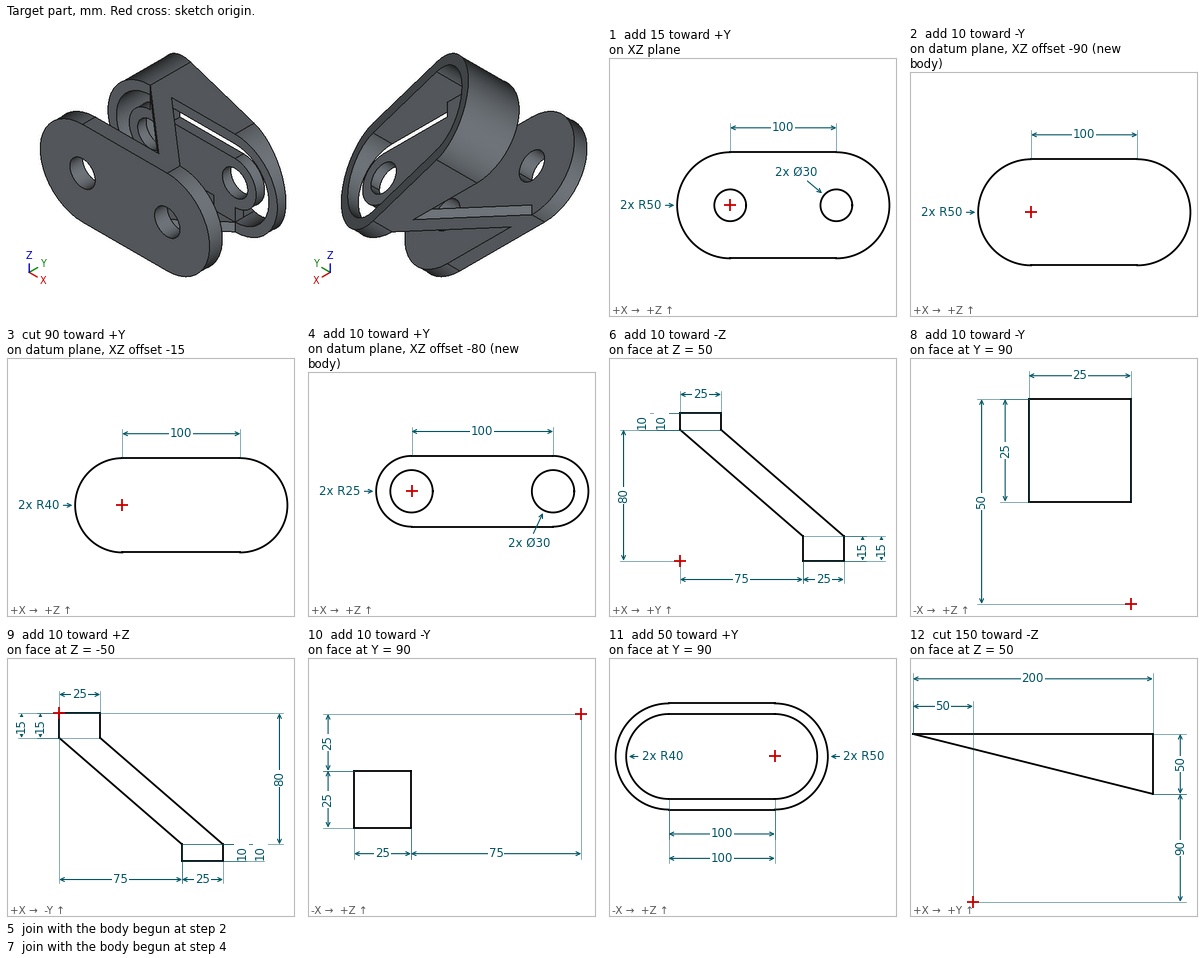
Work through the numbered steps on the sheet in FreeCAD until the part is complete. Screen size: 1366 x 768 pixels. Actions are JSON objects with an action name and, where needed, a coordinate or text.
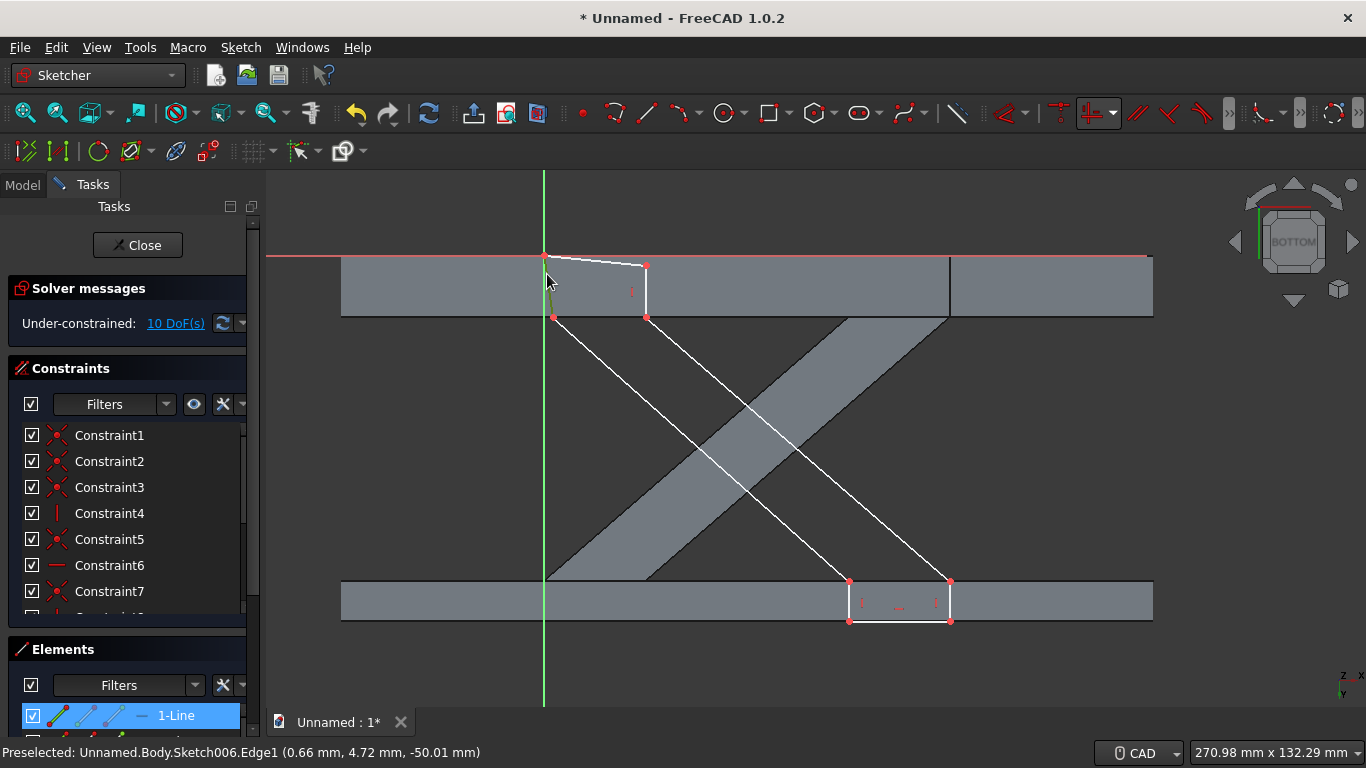
{"action": "left_click", "coordinate": [1116, 114]}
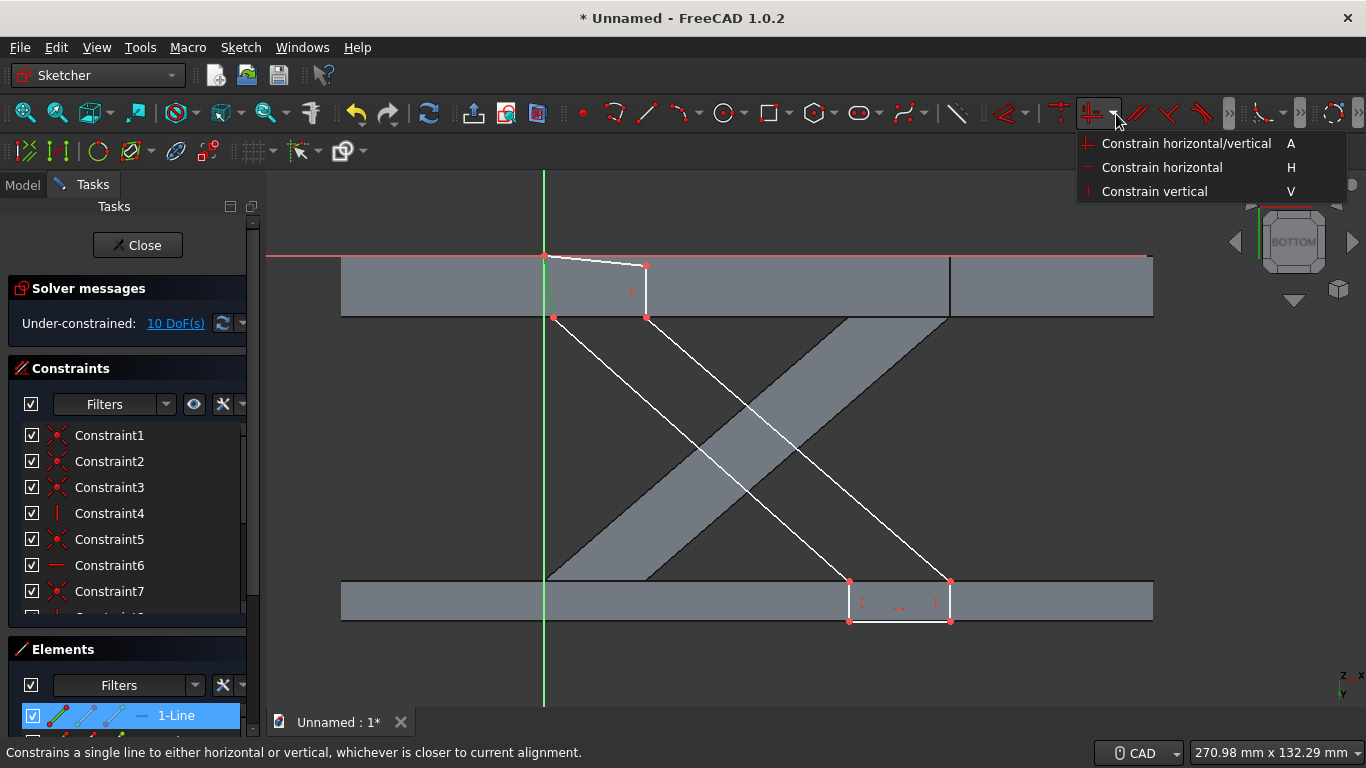
{"action": "left_click", "coordinate": [1212, 191]}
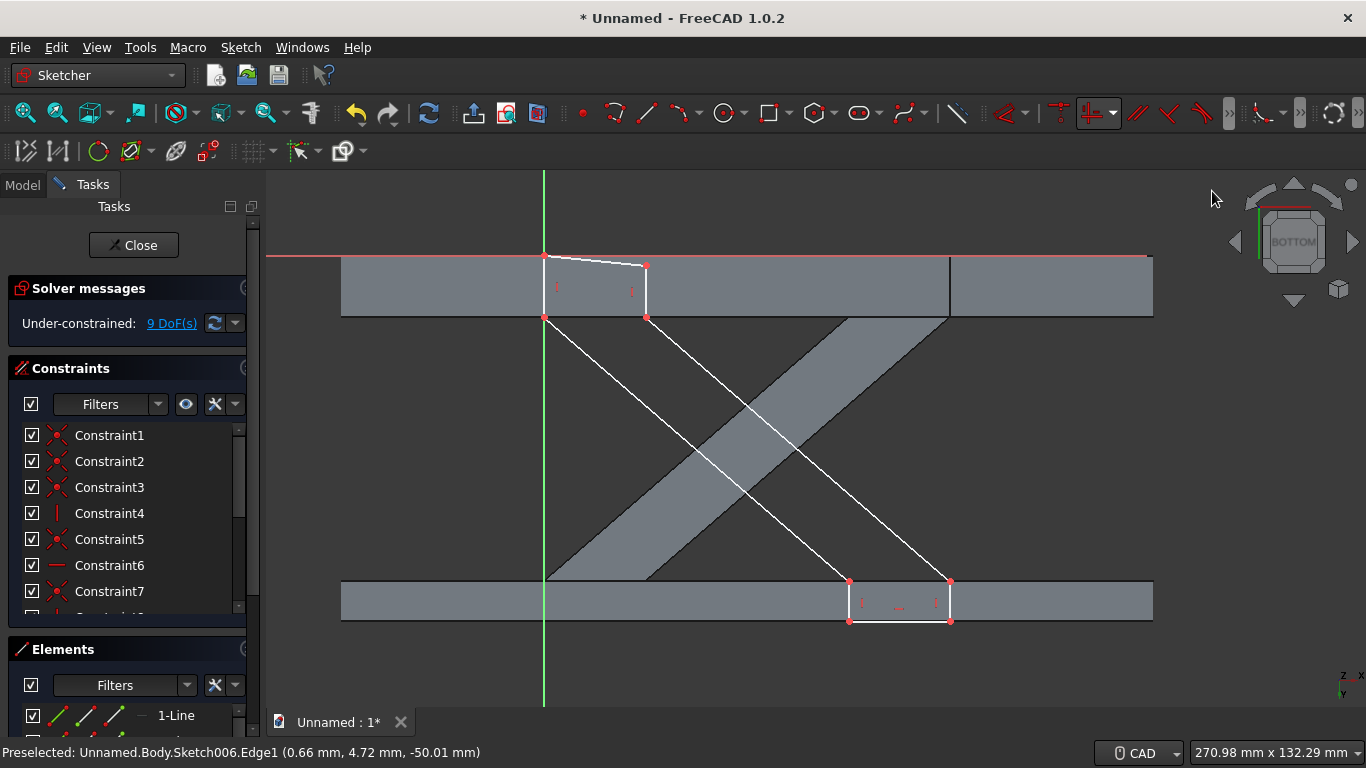
{"action": "left_click", "coordinate": [575, 259]}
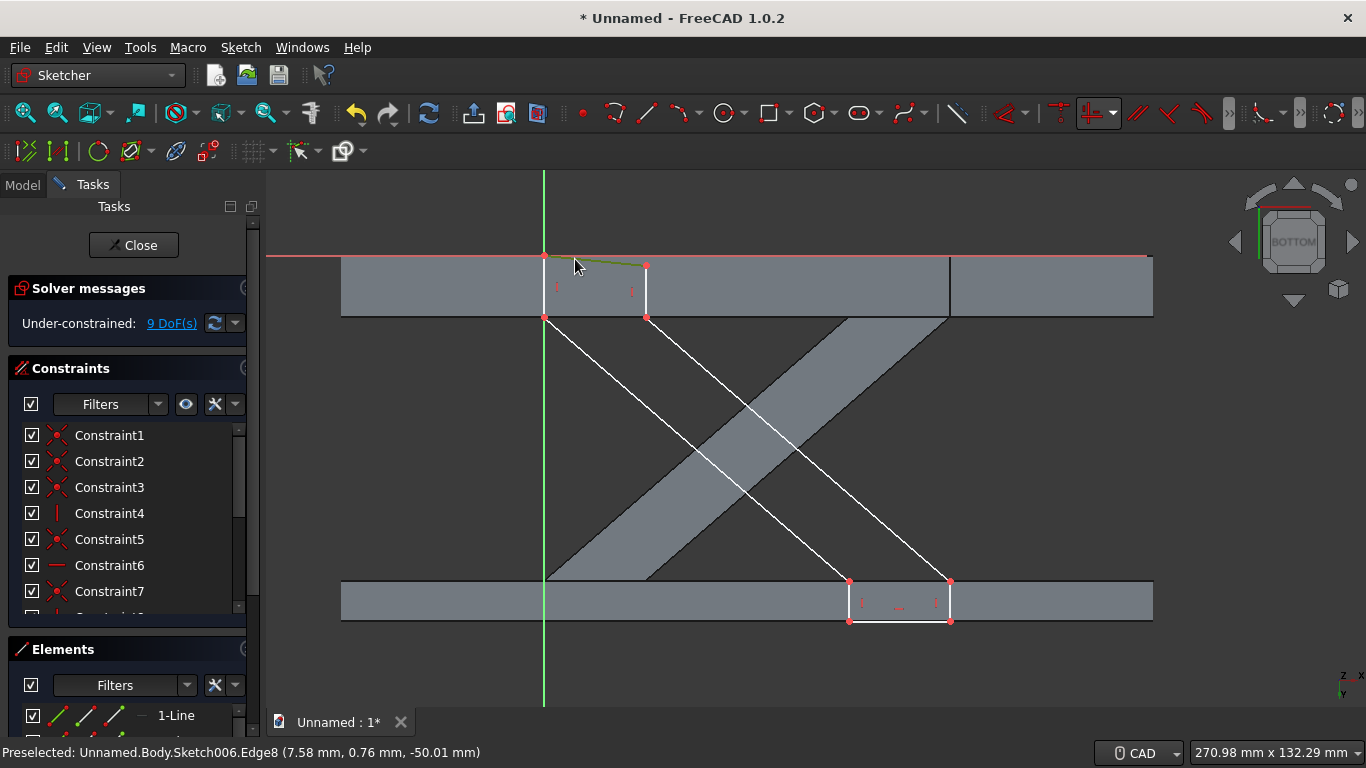
{"action": "left_click", "coordinate": [1116, 114]}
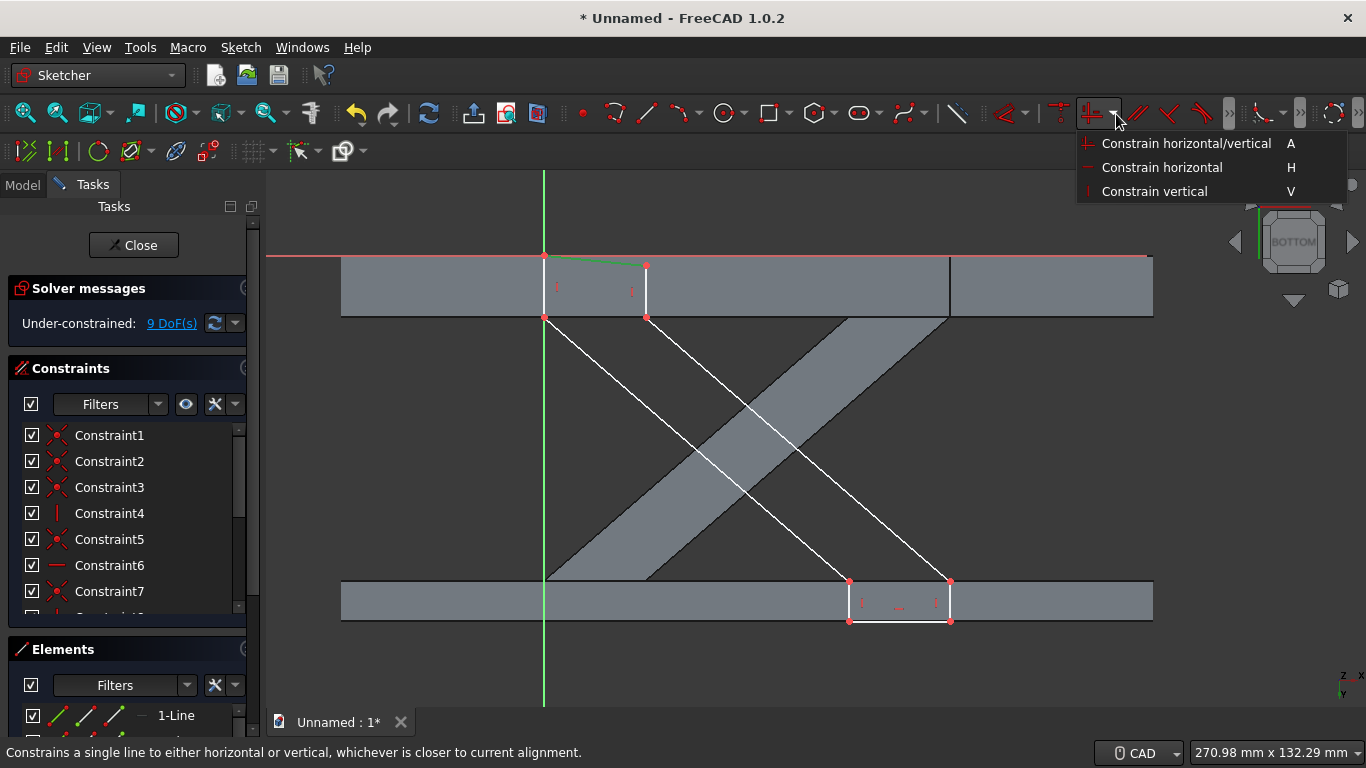
{"action": "left_click", "coordinate": [1212, 167]}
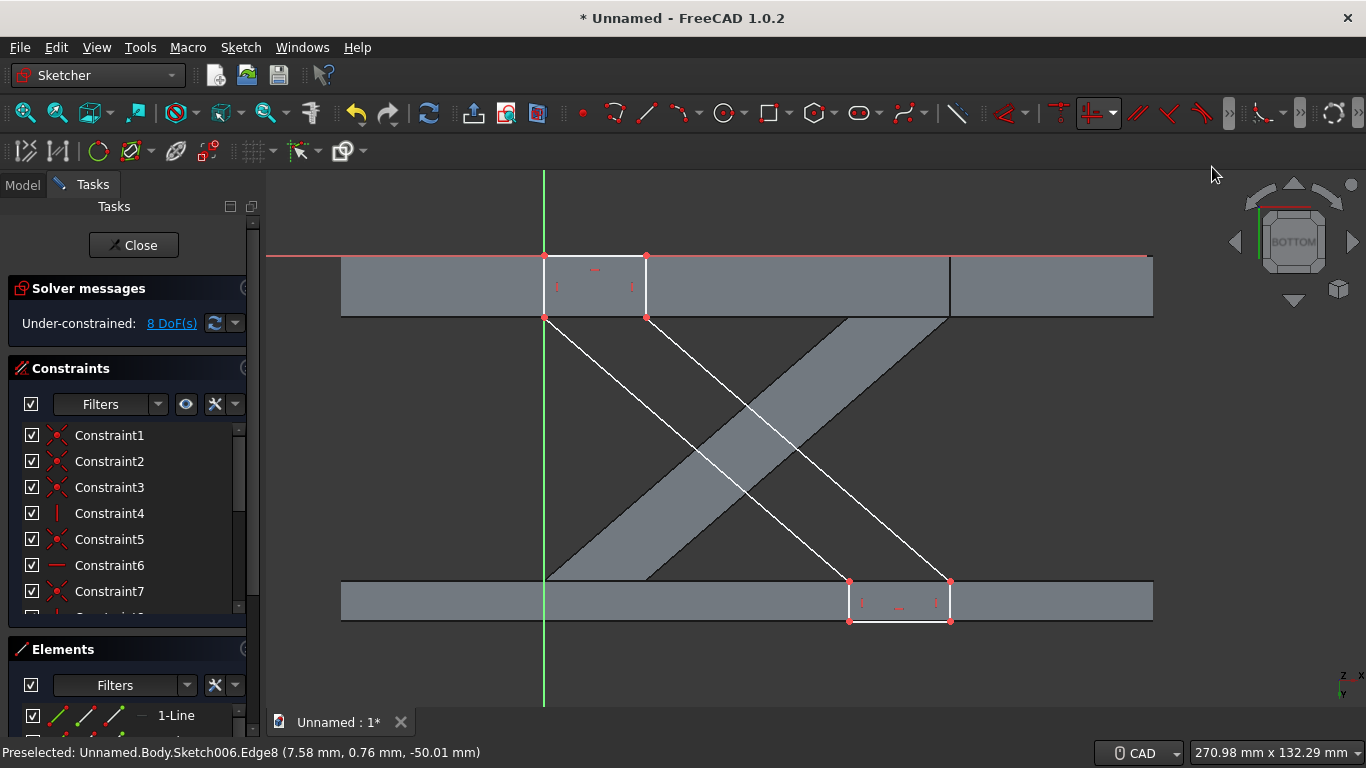
{"action": "left_click", "coordinate": [1004, 114]}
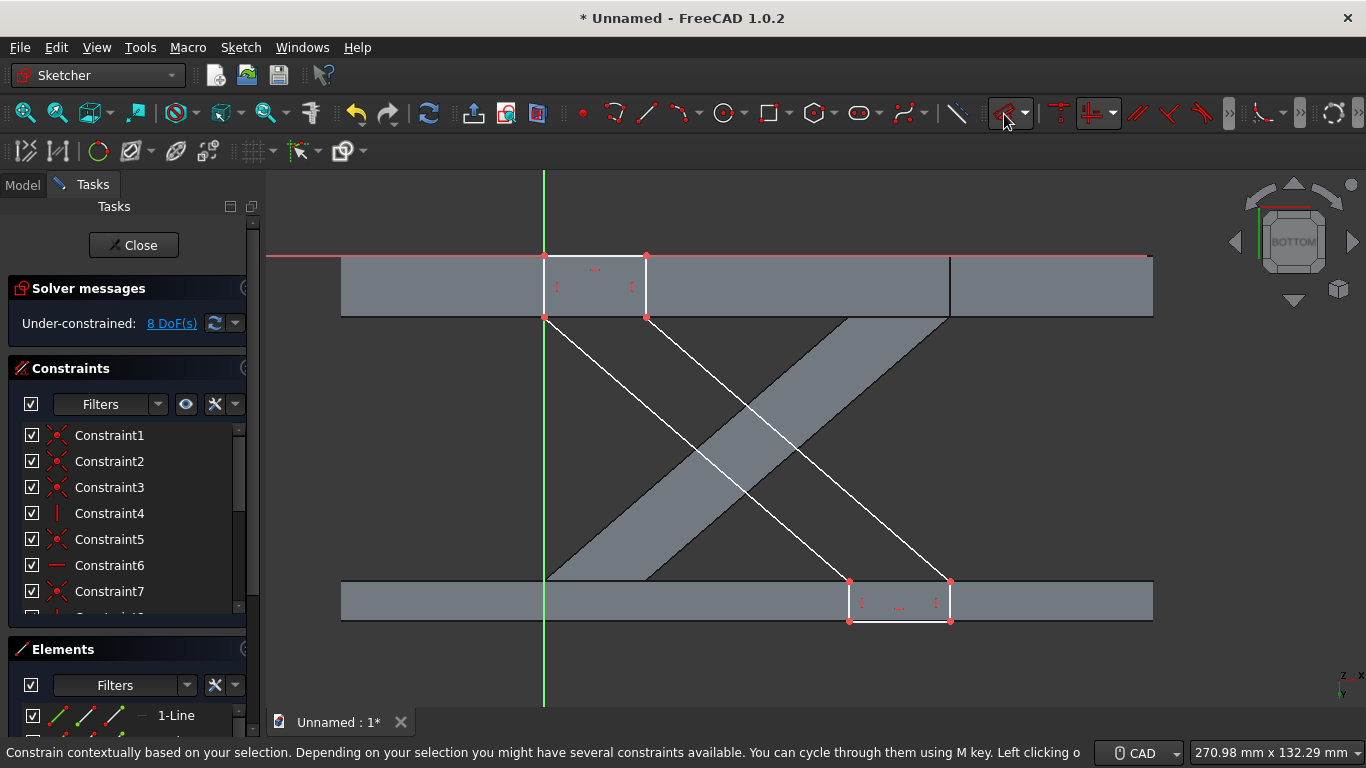
{"action": "left_click", "coordinate": [544, 274]}
{"action": "left_click", "coordinate": [510, 287]}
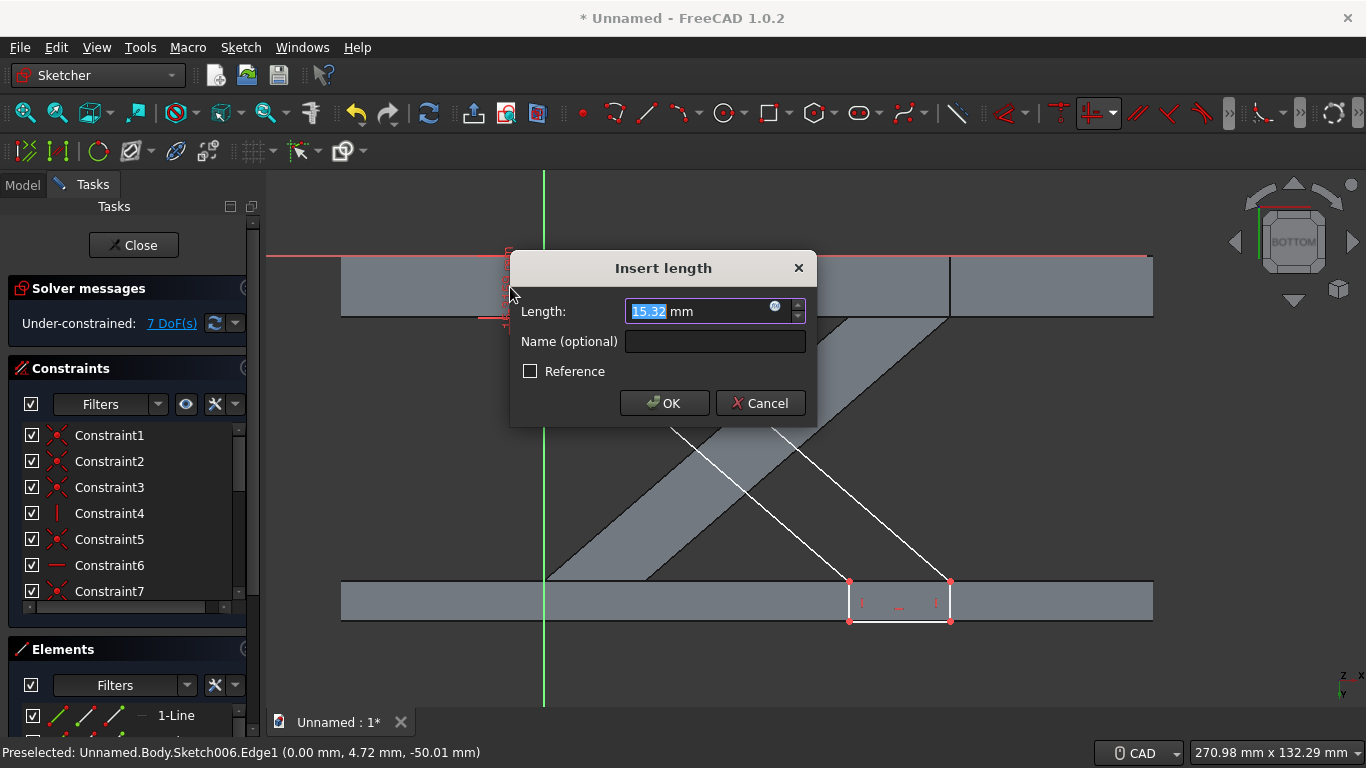
{"action": "type", "text": "15"}
{"action": "key", "text": "Return"}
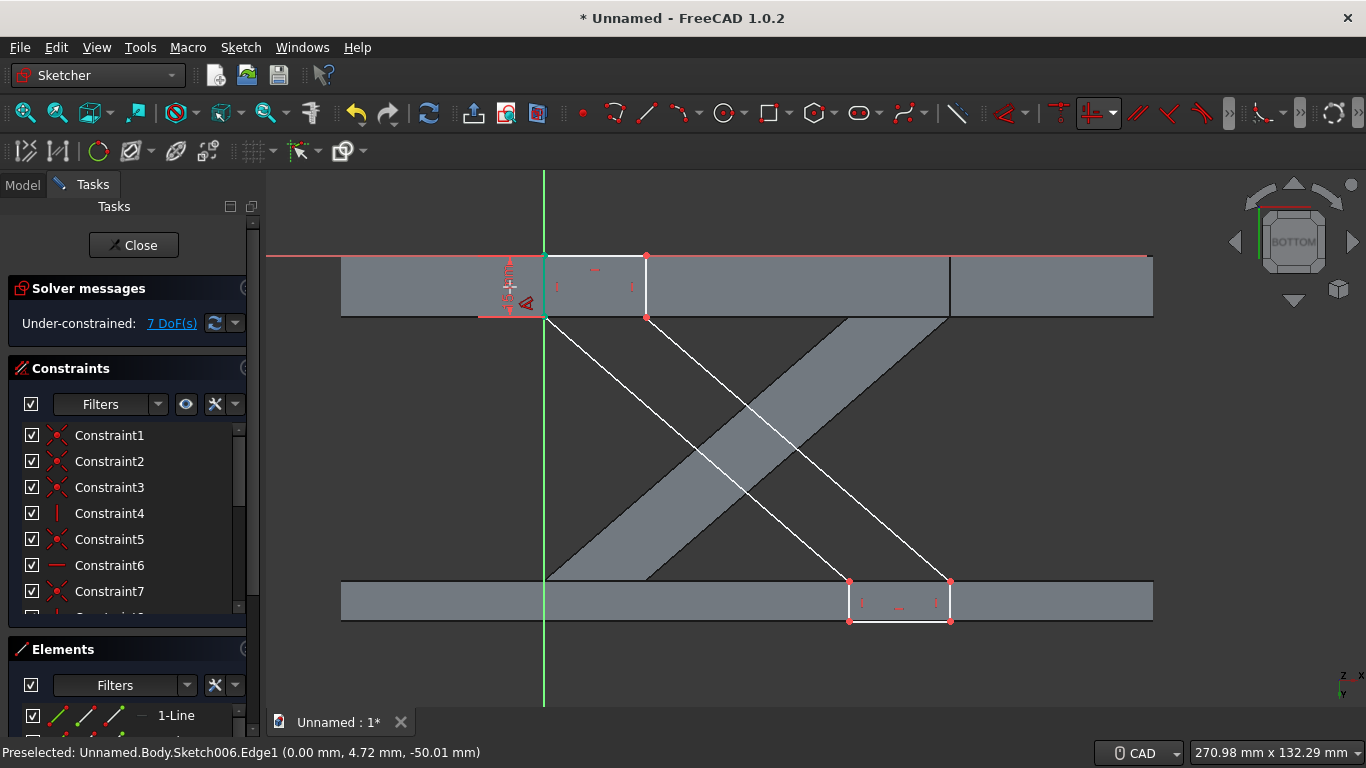
{"action": "left_click", "coordinate": [849, 594]}
{"action": "left_click", "coordinate": [883, 602]}